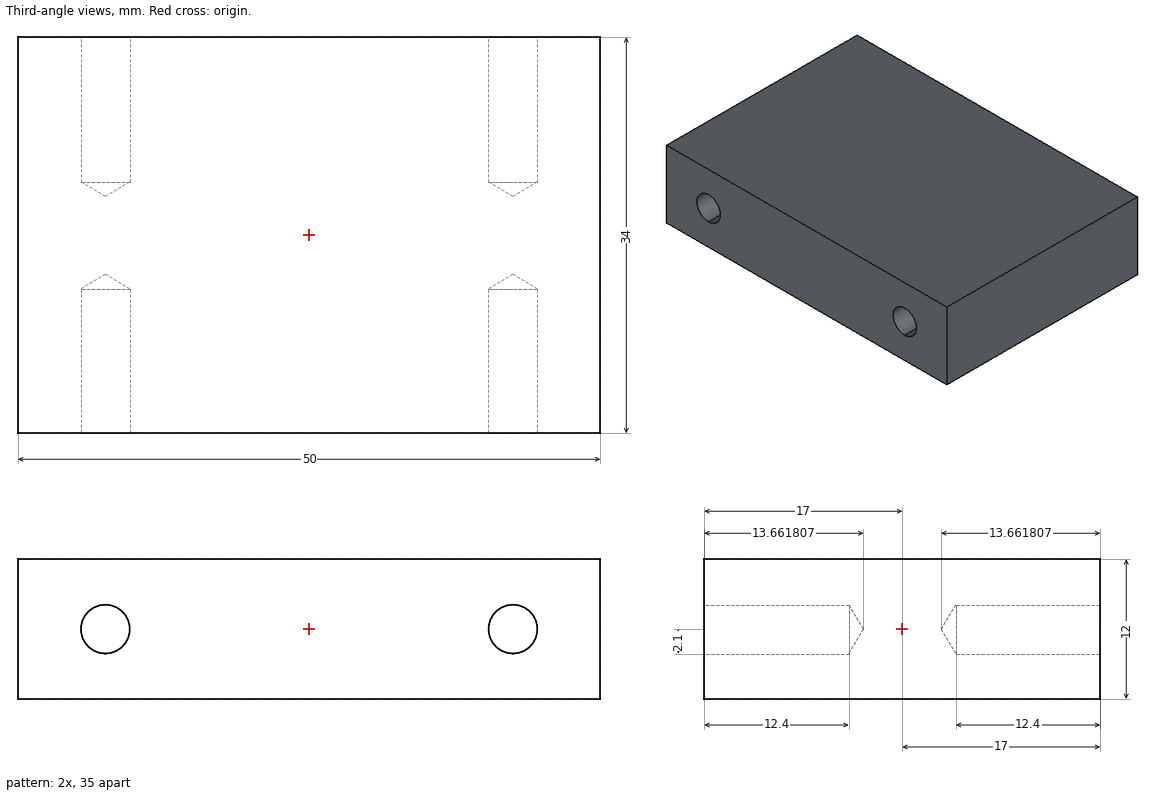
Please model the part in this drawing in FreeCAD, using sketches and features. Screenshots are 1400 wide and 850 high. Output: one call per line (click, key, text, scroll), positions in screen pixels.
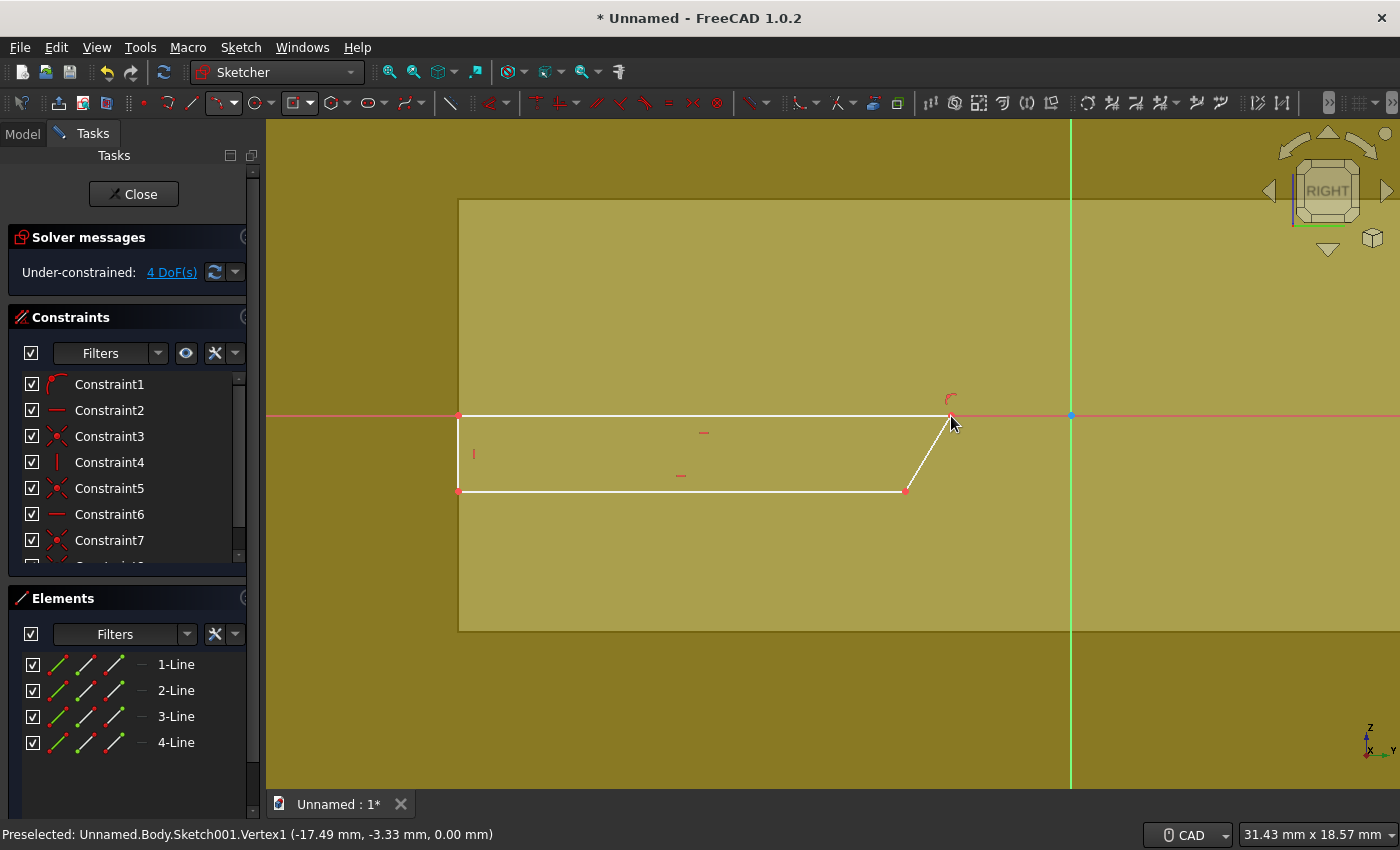
click(458, 439)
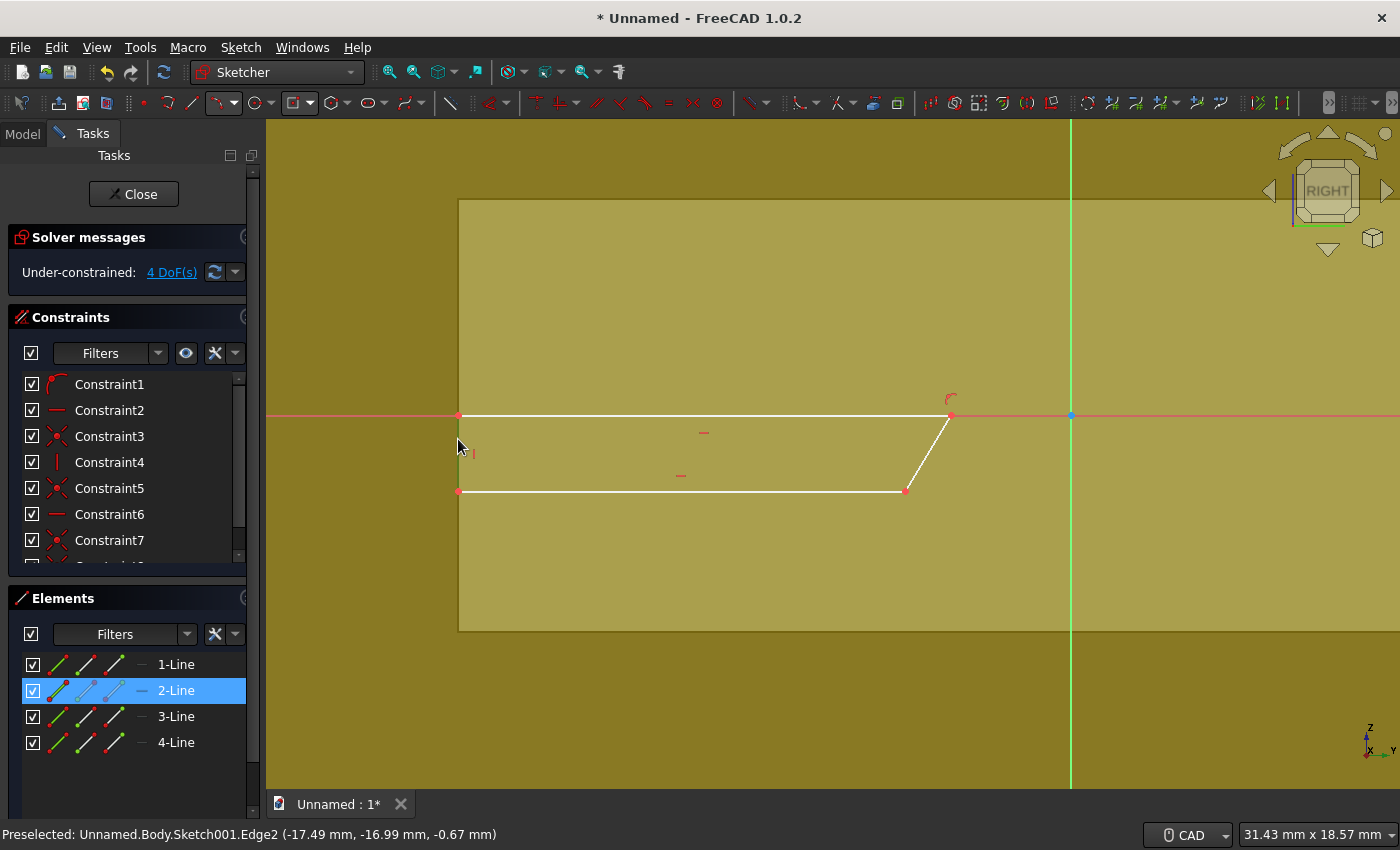
key(i)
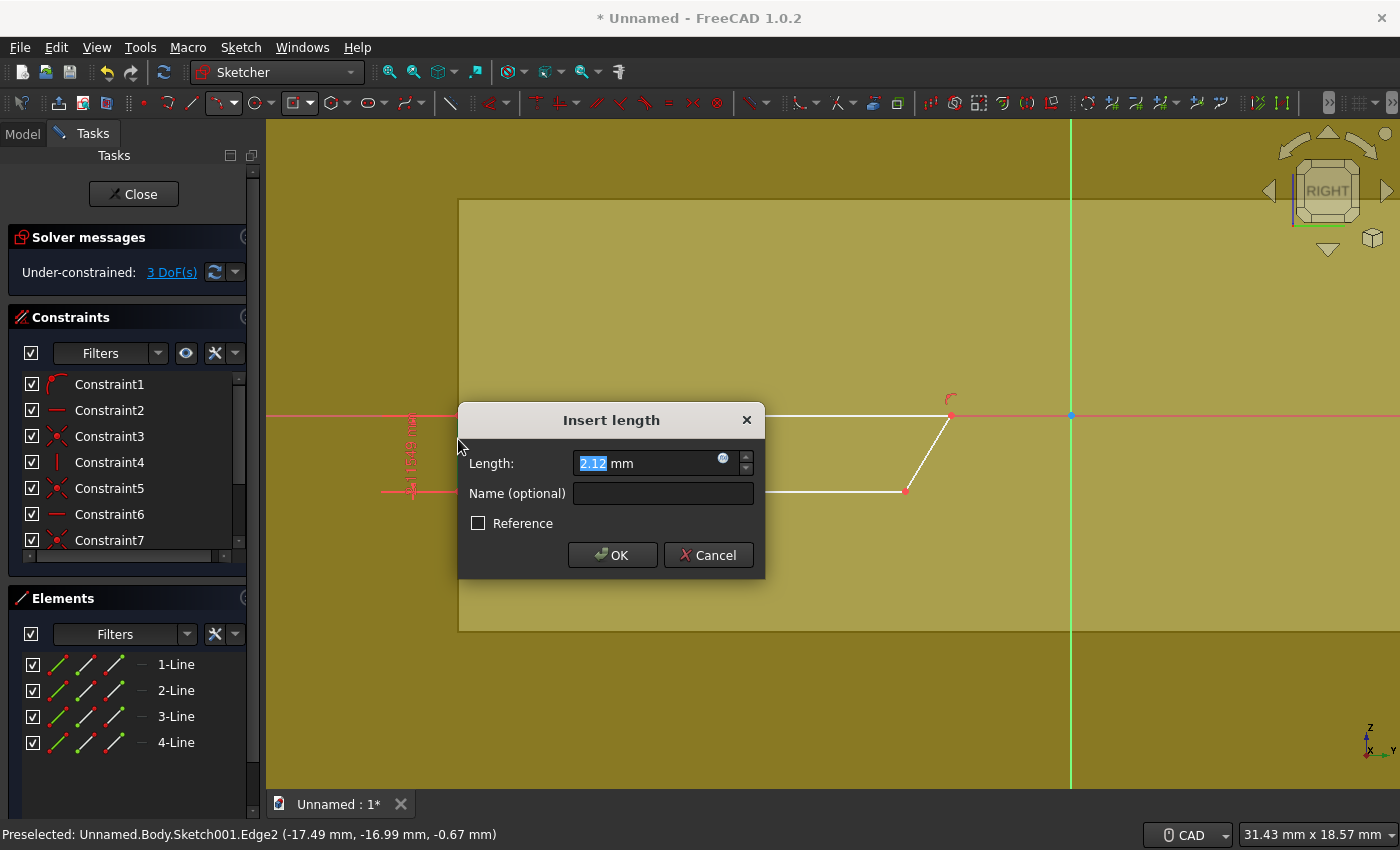
text(2.1)
key(Return)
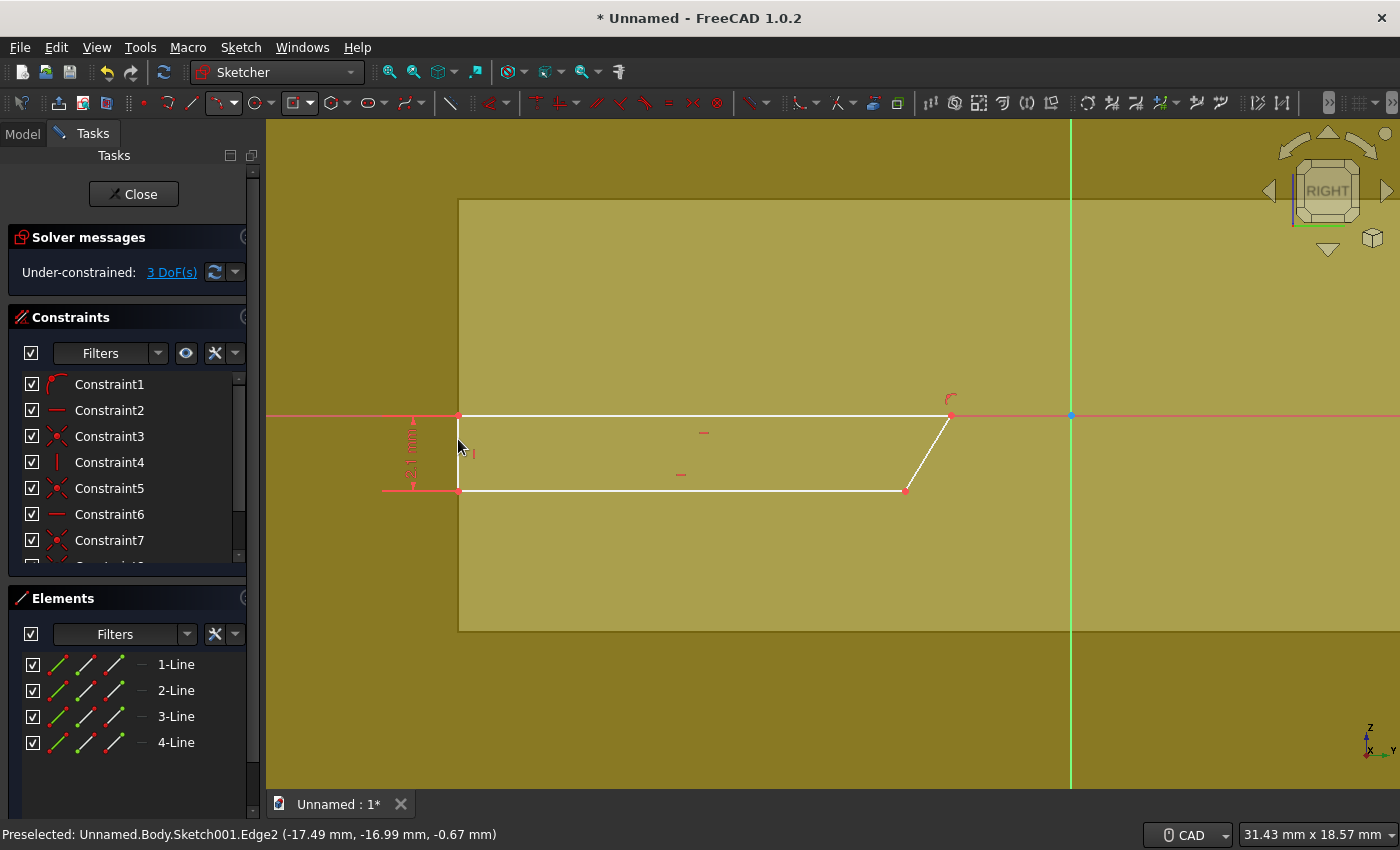
click(458, 416)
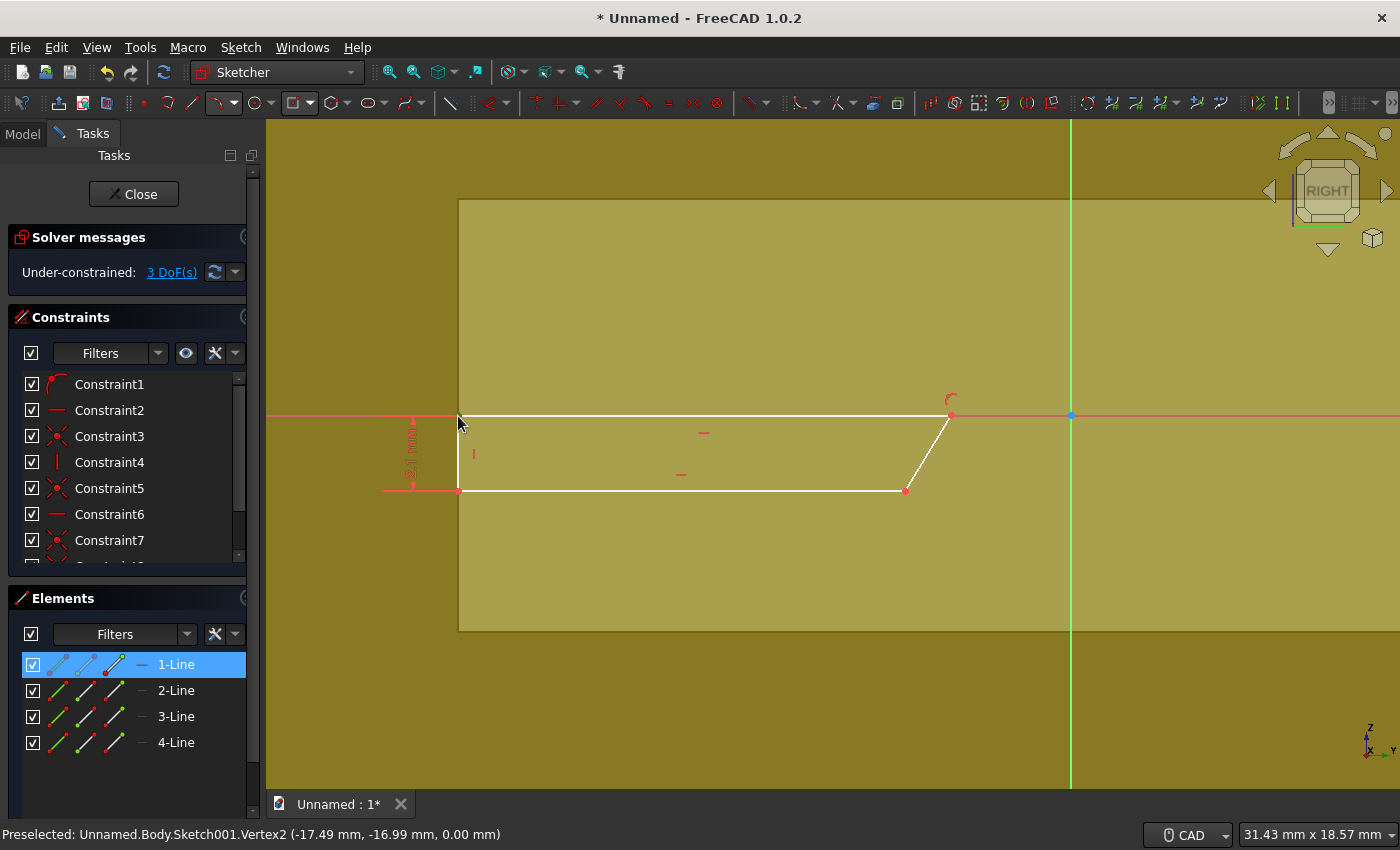
key(l)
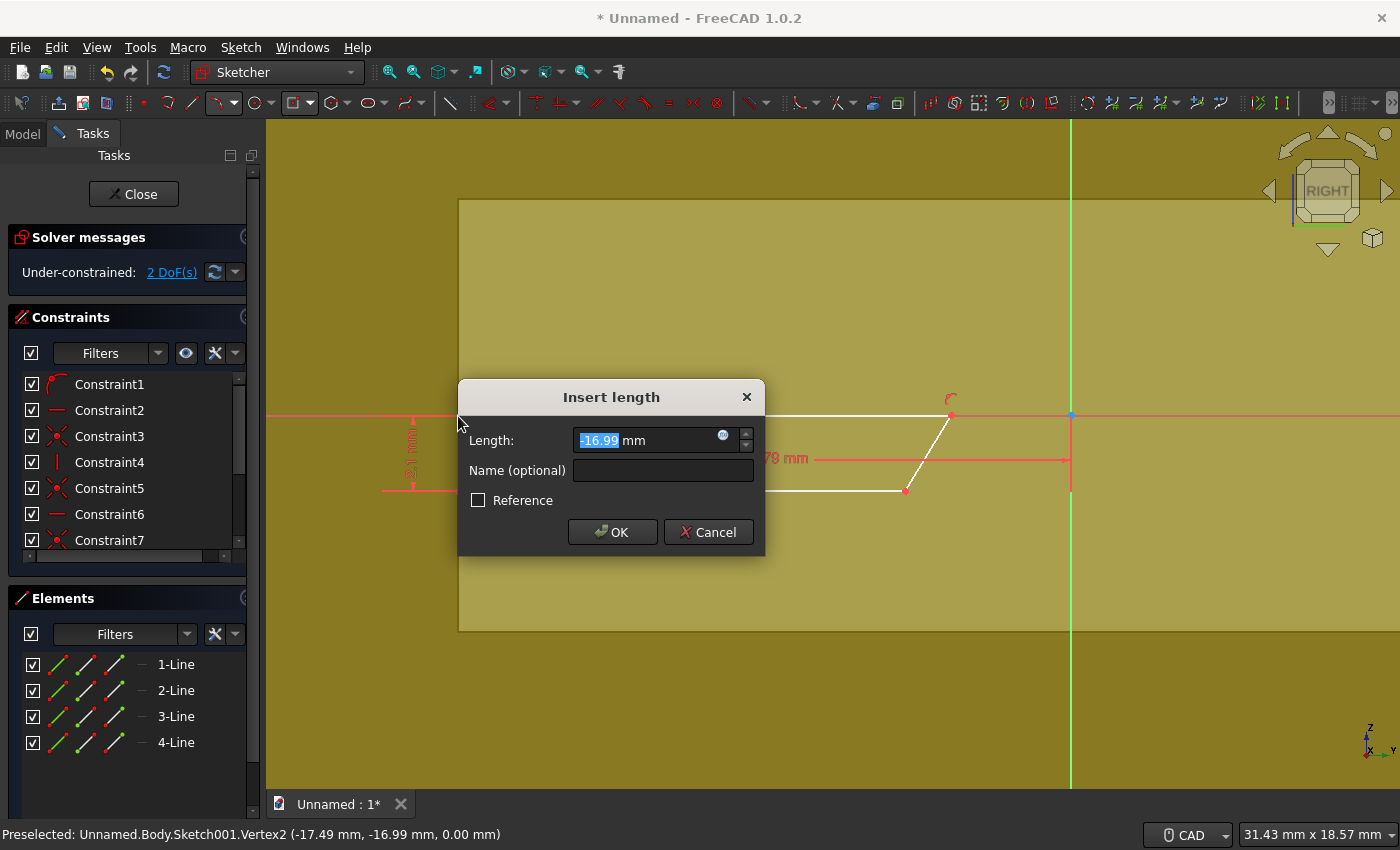
text(-17)
key(Return)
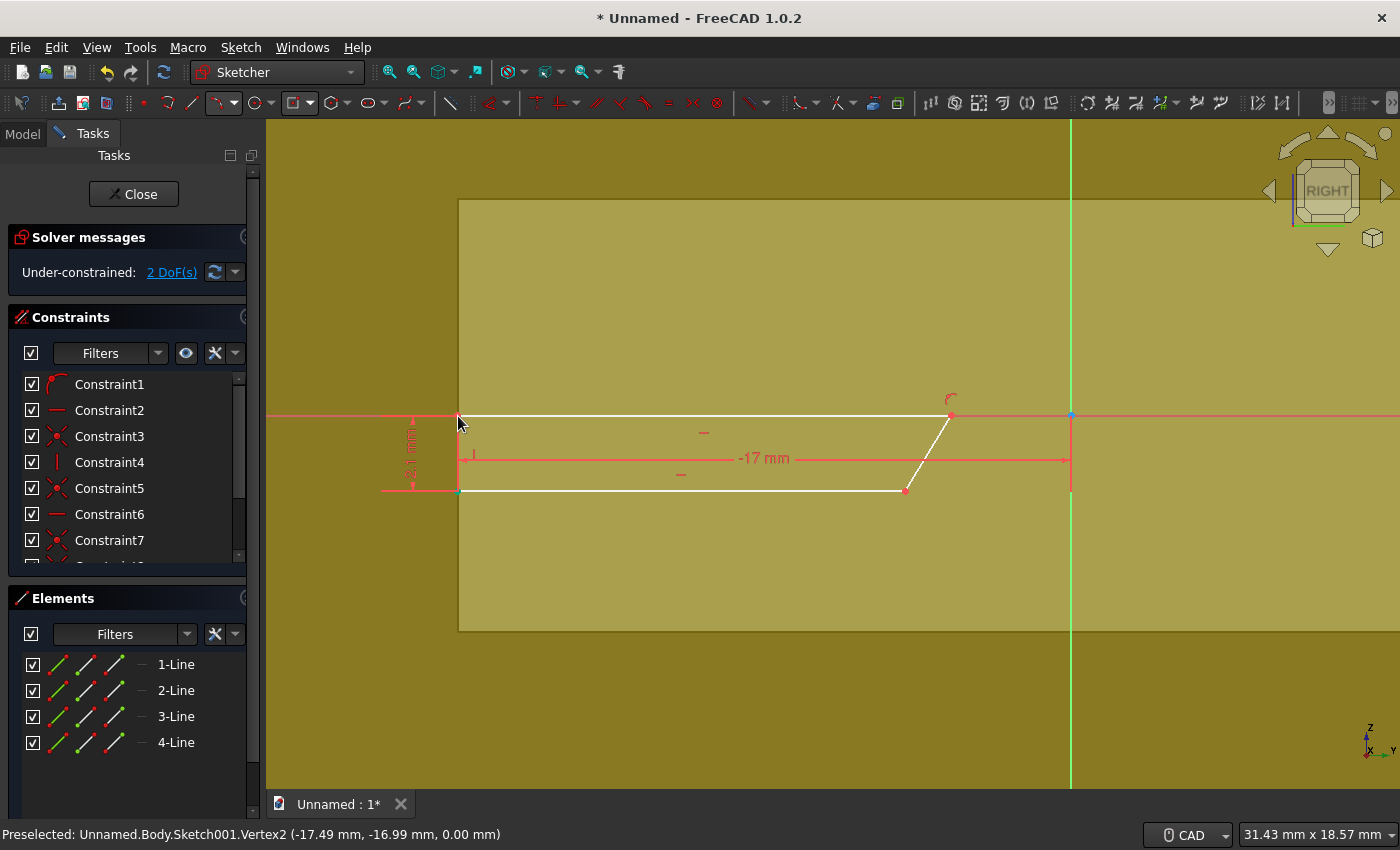
click(592, 491)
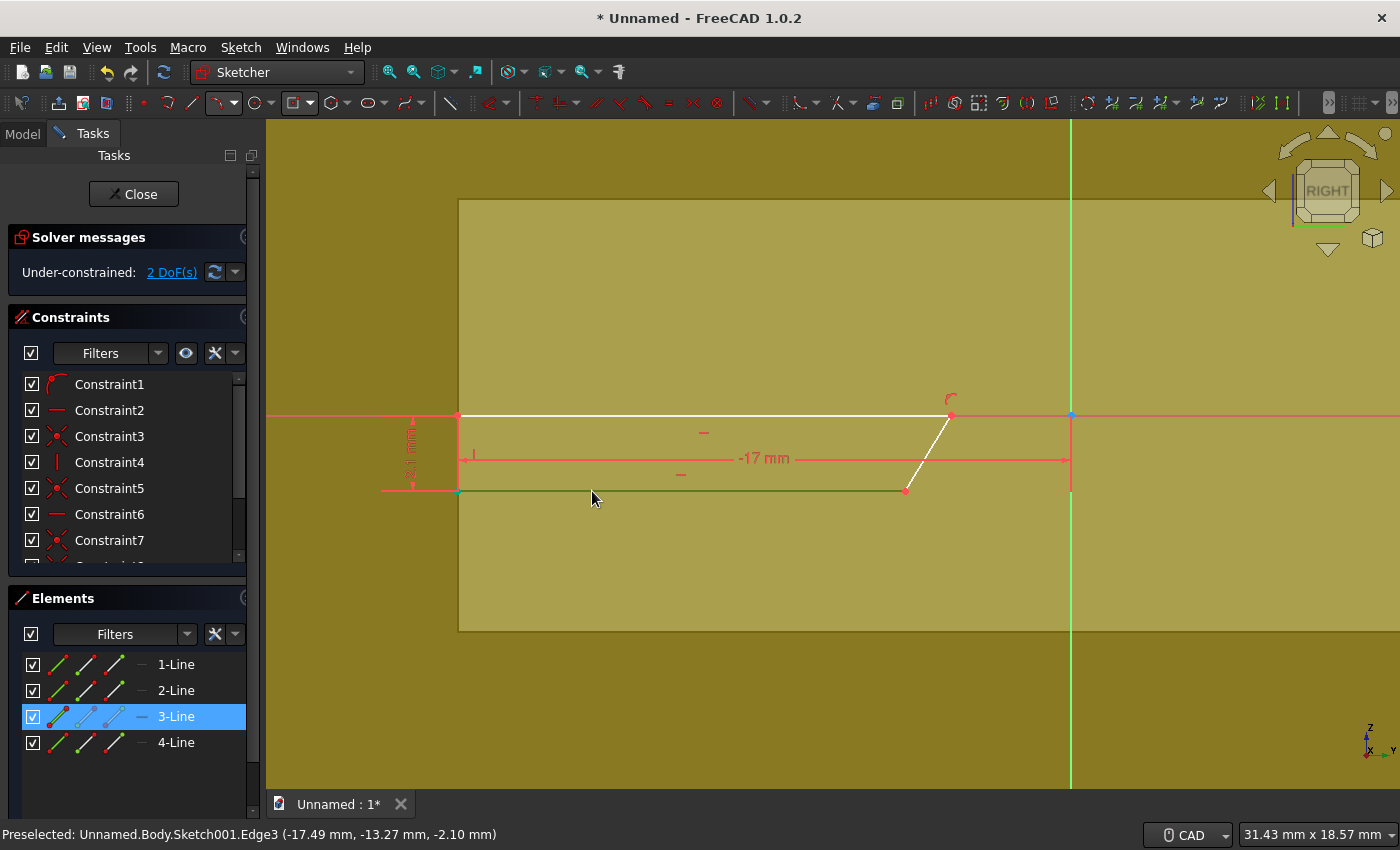
click(508, 104)